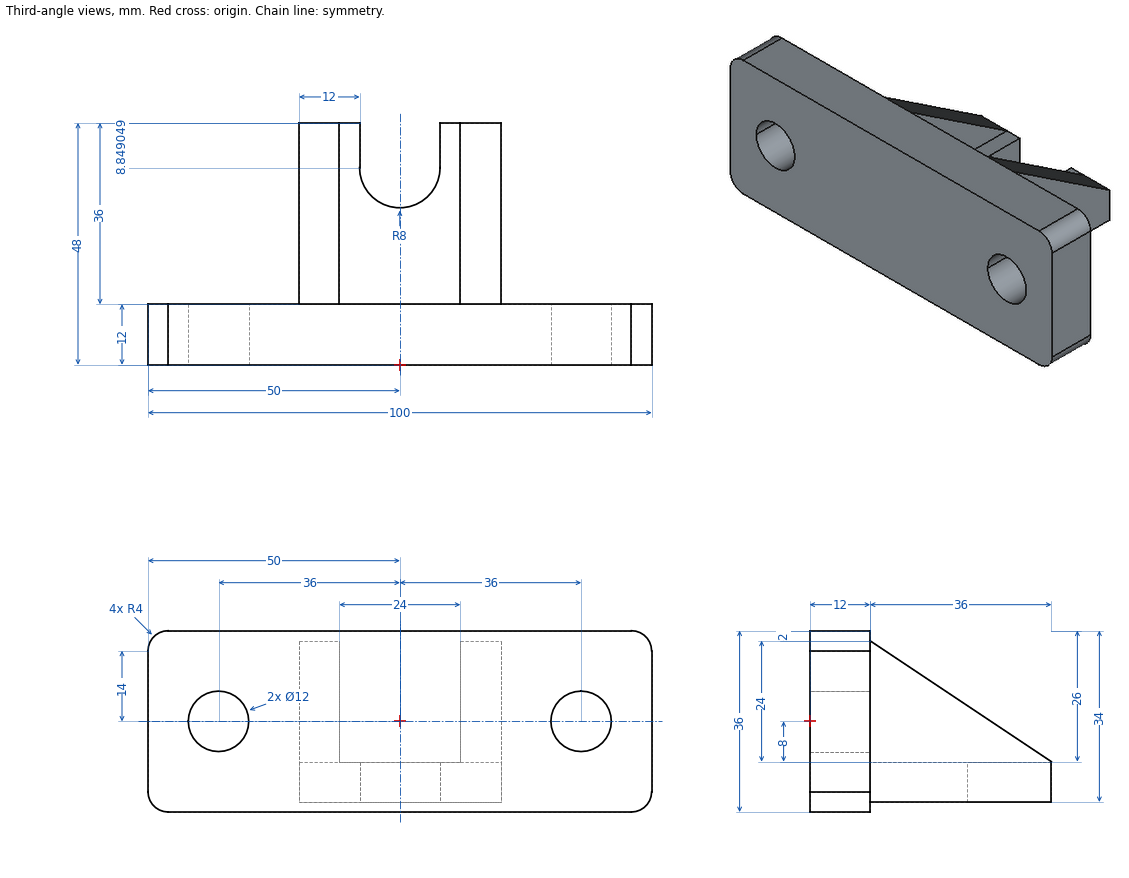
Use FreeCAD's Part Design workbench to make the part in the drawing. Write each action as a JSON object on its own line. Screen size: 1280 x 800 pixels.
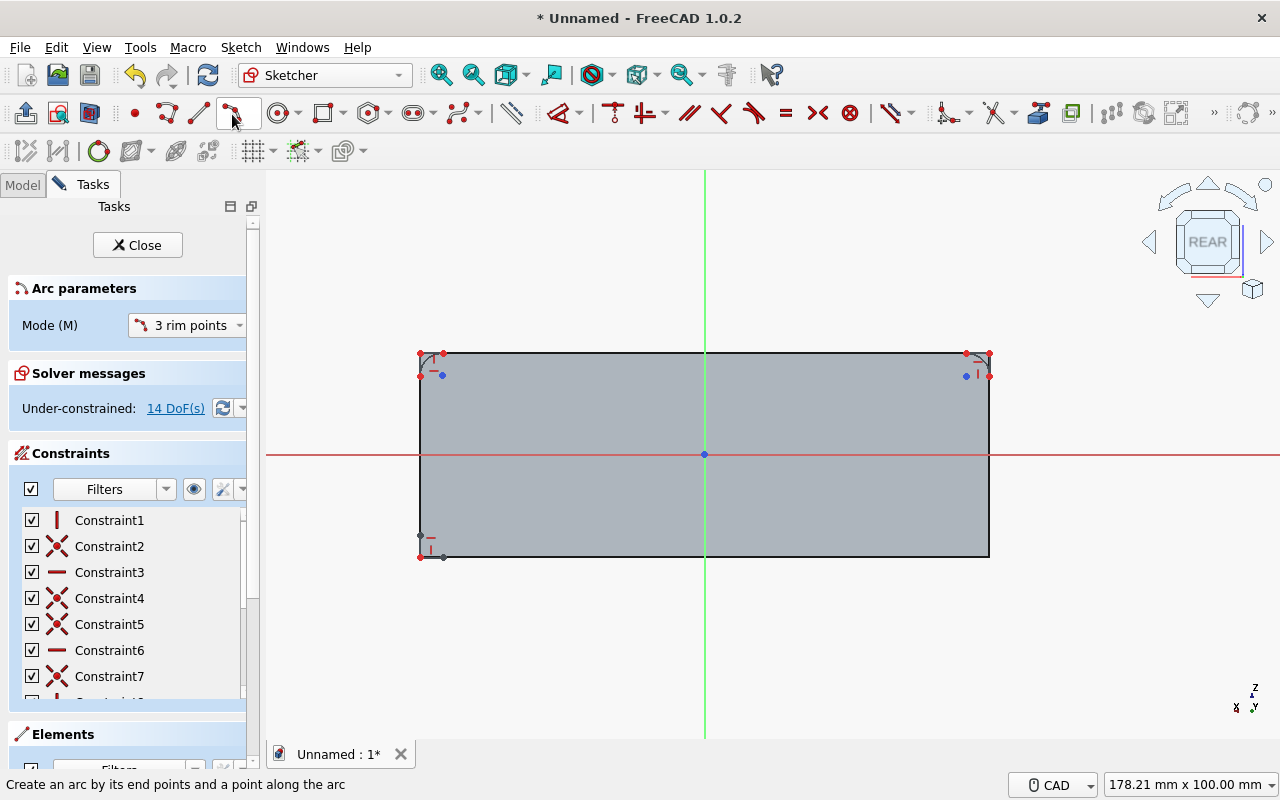
{"action": "scroll", "coordinate": [443, 557], "scroll_direction": "up", "scroll_amount": 2}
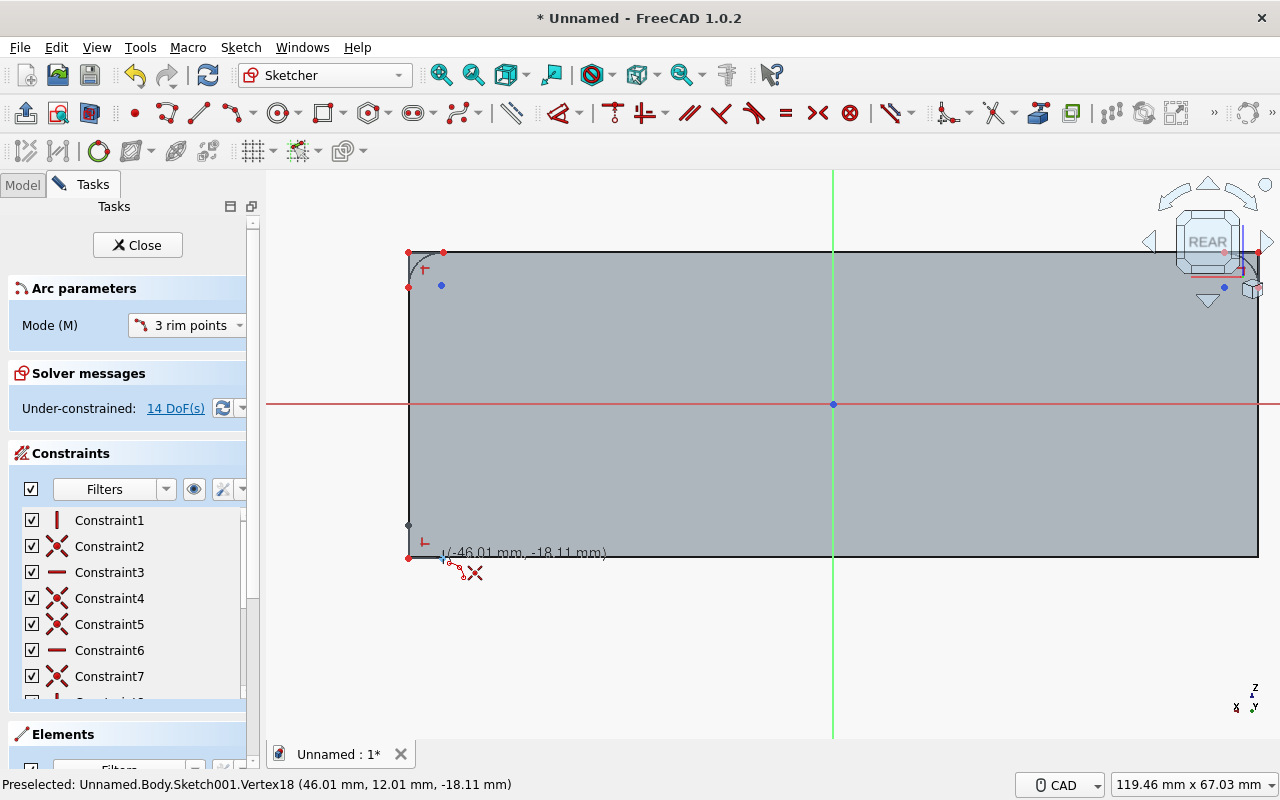
{"action": "left_click", "coordinate": [443, 558]}
{"action": "left_click", "coordinate": [409, 525]}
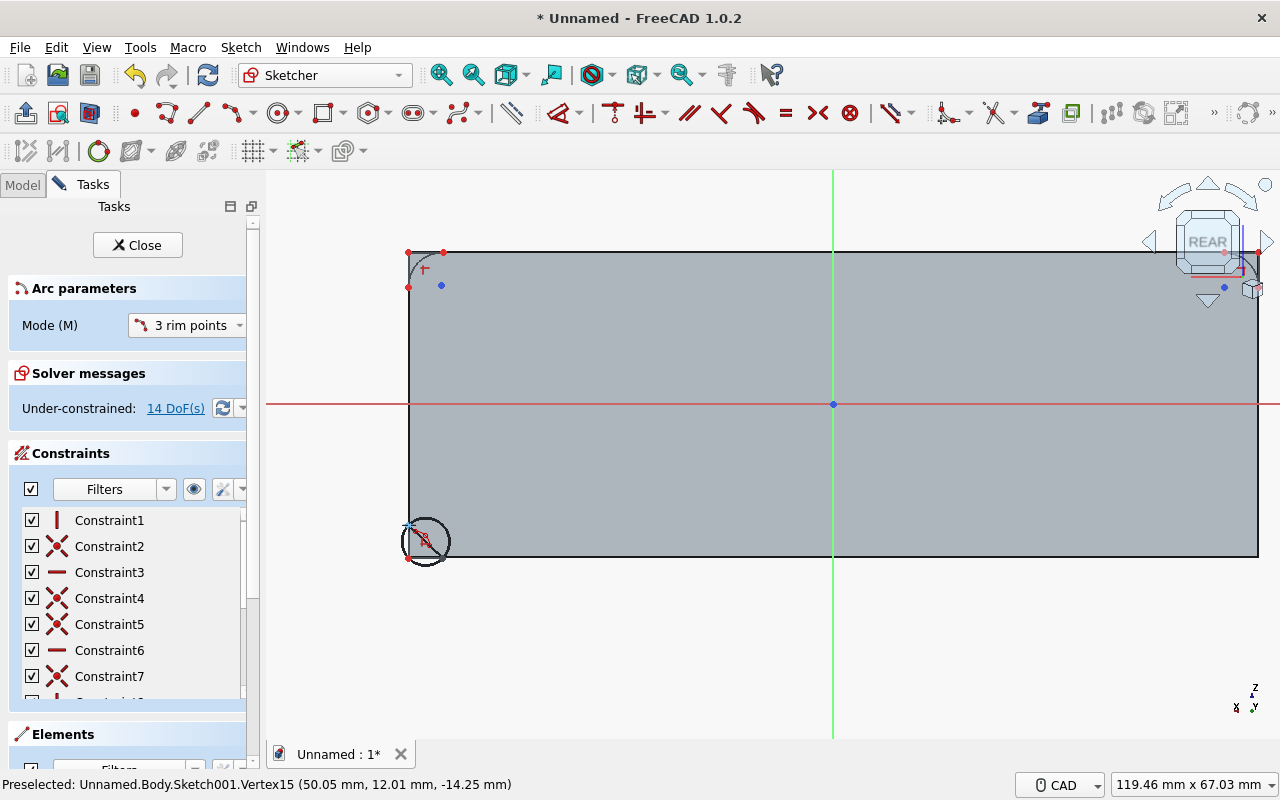
{"action": "scroll", "coordinate": [419, 547], "scroll_direction": "up", "scroll_amount": 3}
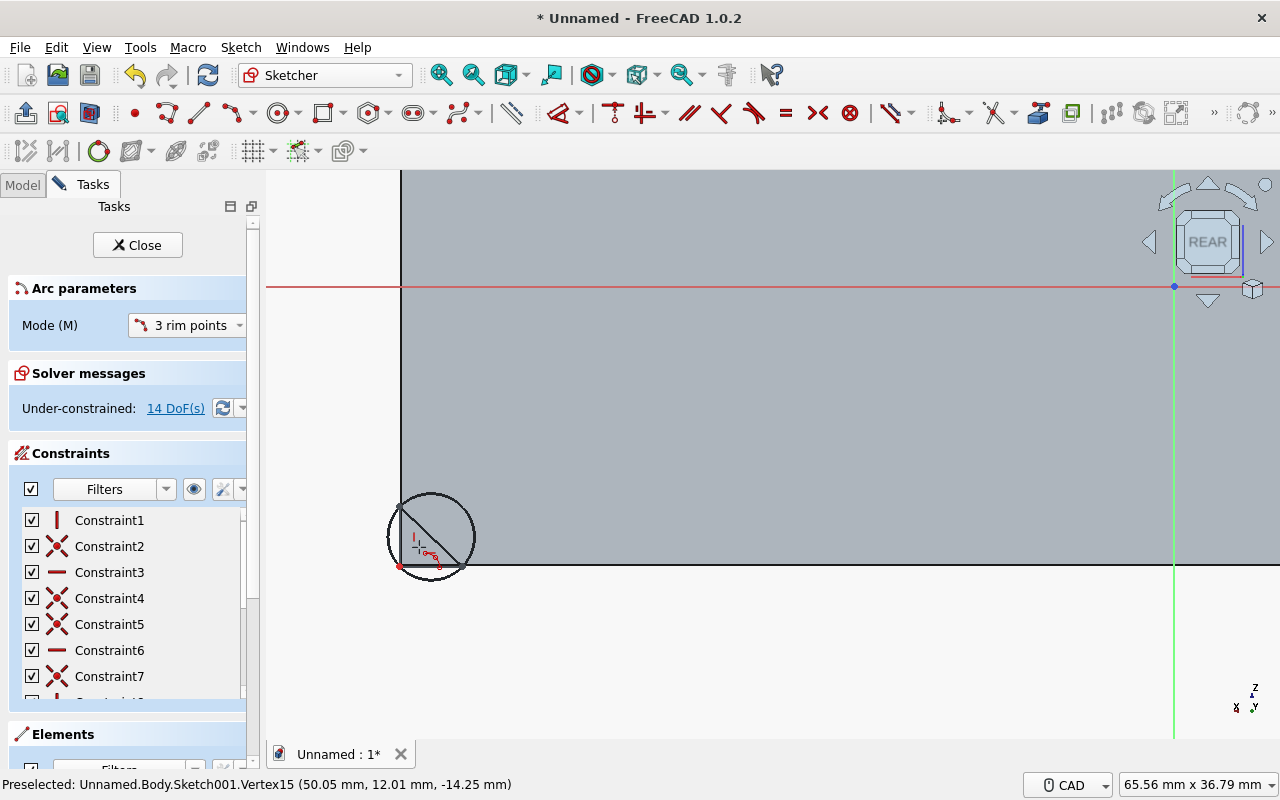
{"action": "left_click", "coordinate": [419, 547]}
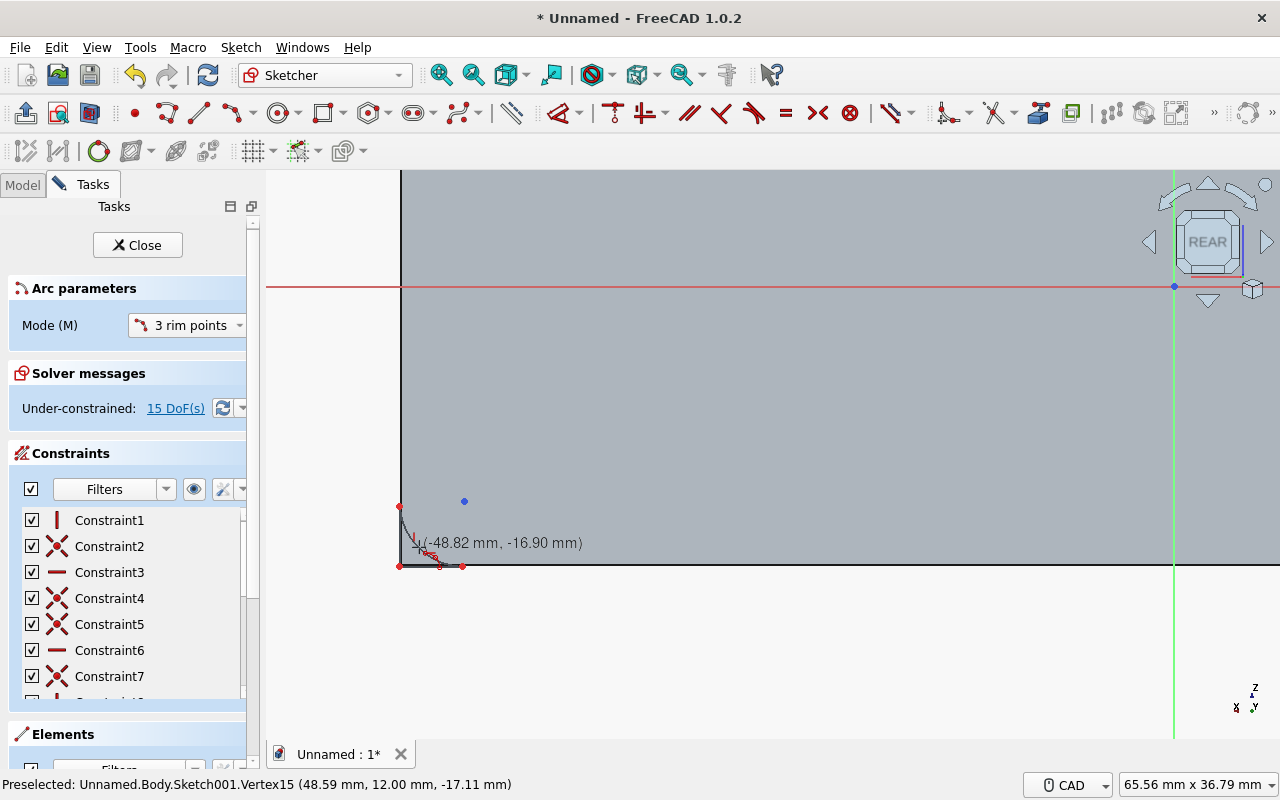
{"action": "left_click", "coordinate": [168, 114]}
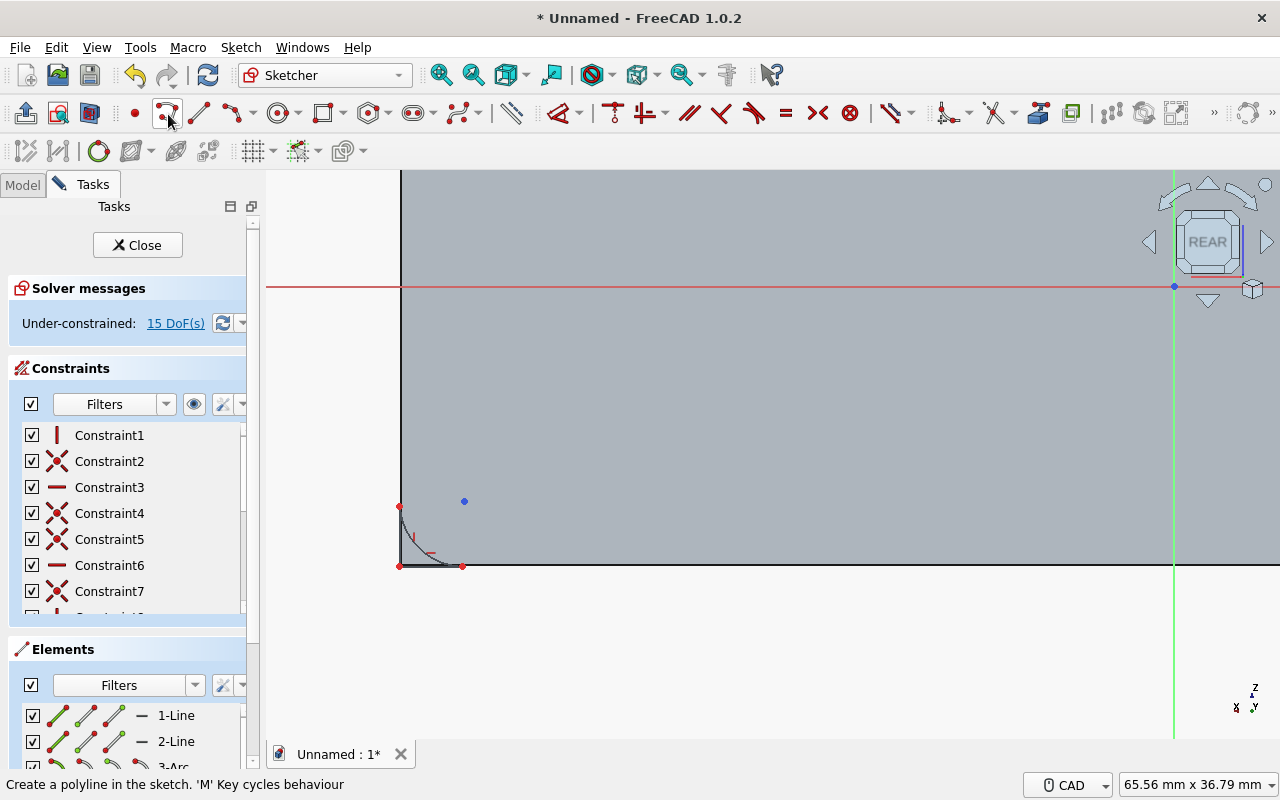
{"action": "scroll", "coordinate": [431, 552], "scroll_direction": "down", "scroll_amount": 5}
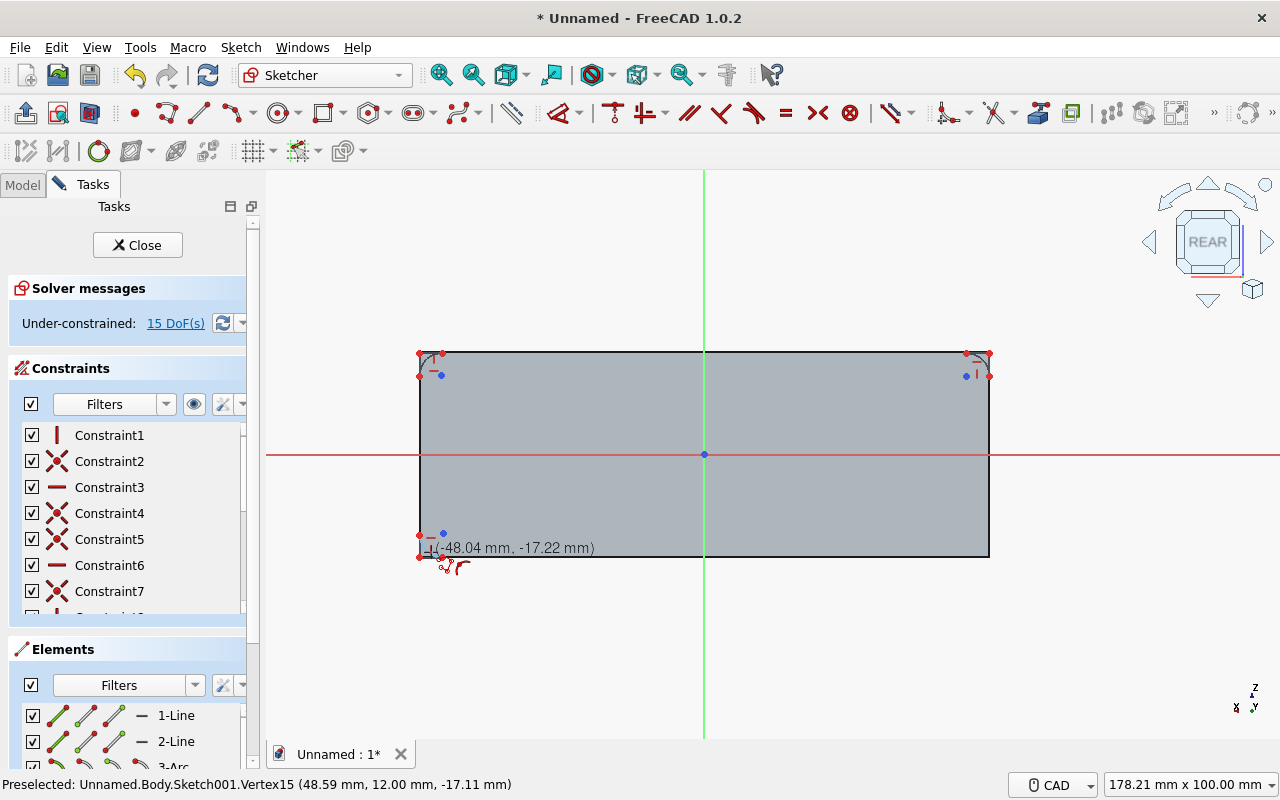
{"action": "left_click", "coordinate": [966, 557]}
{"action": "left_click", "coordinate": [989, 557]}
{"action": "left_click", "coordinate": [989, 534]}
{"action": "right_click", "coordinate": [989, 534]}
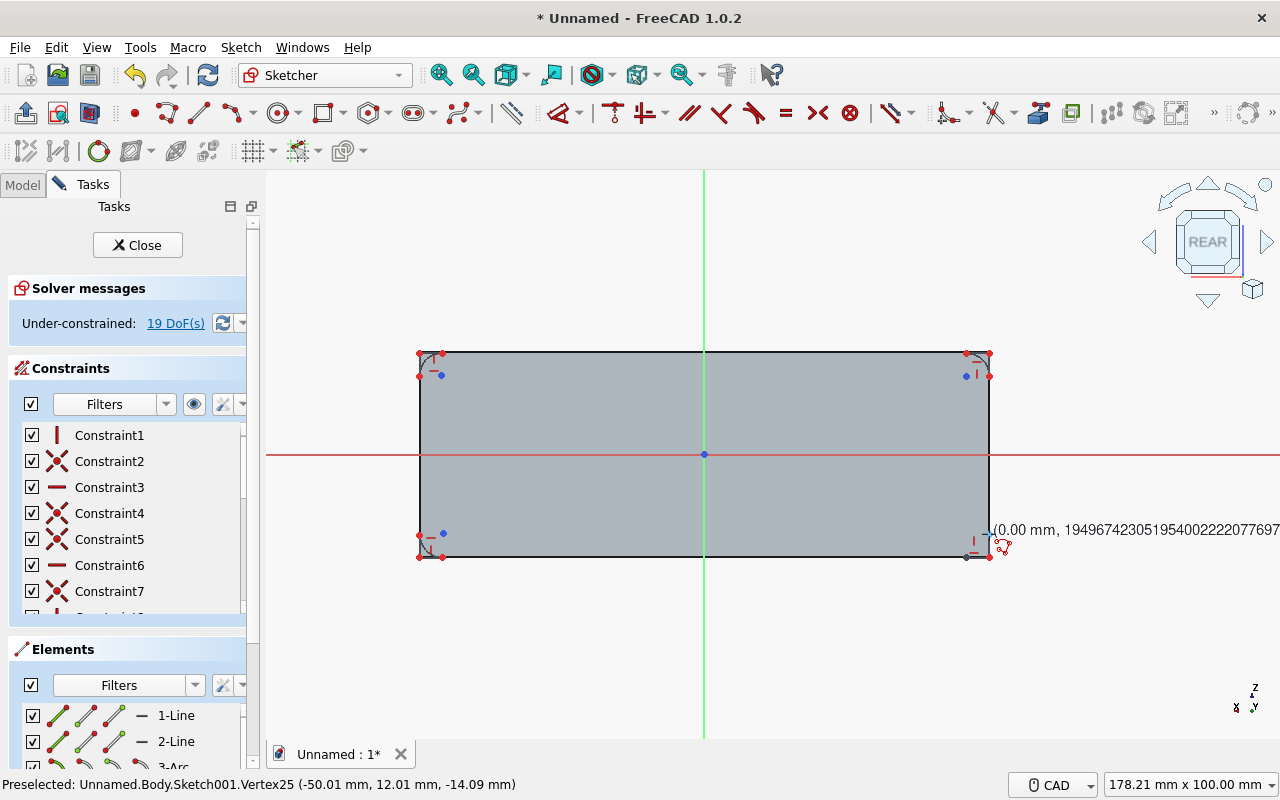
{"action": "left_click", "coordinate": [232, 114]}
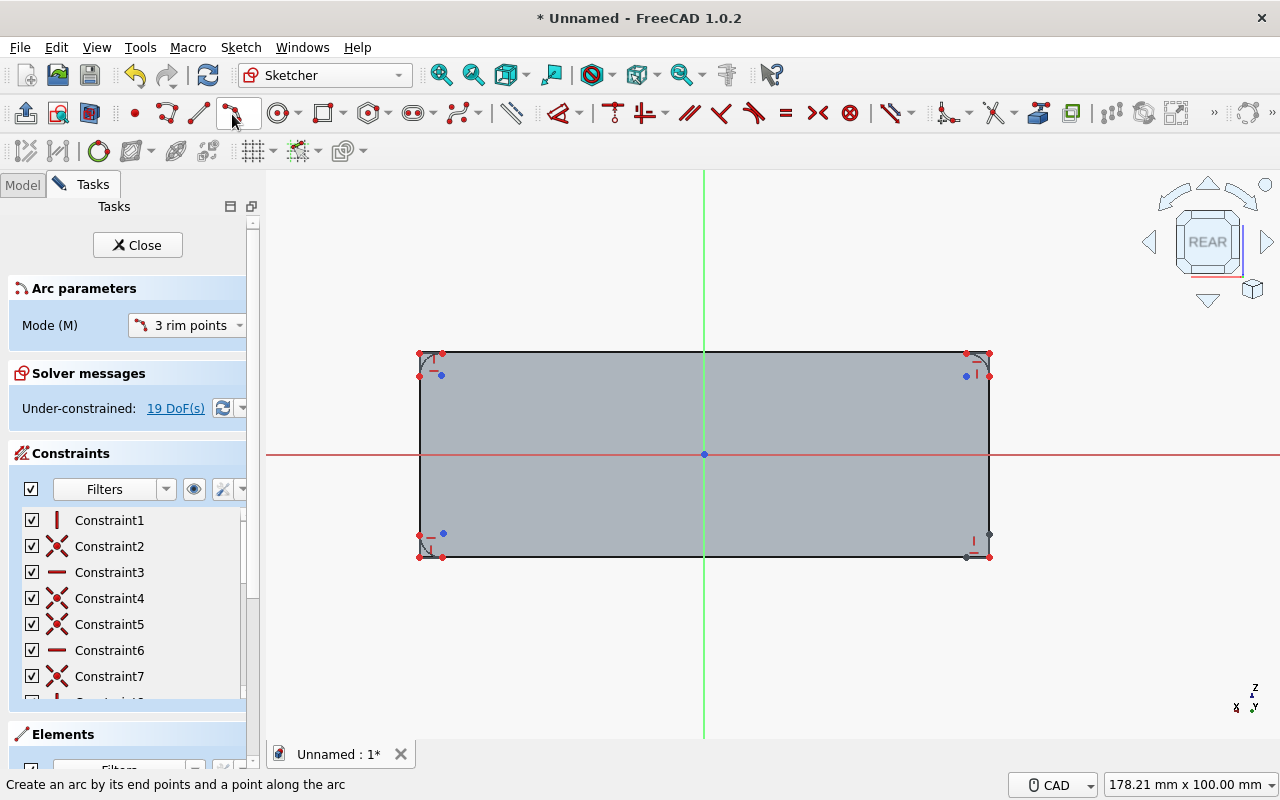
{"action": "scroll", "coordinate": [989, 534], "scroll_direction": "up", "scroll_amount": 2}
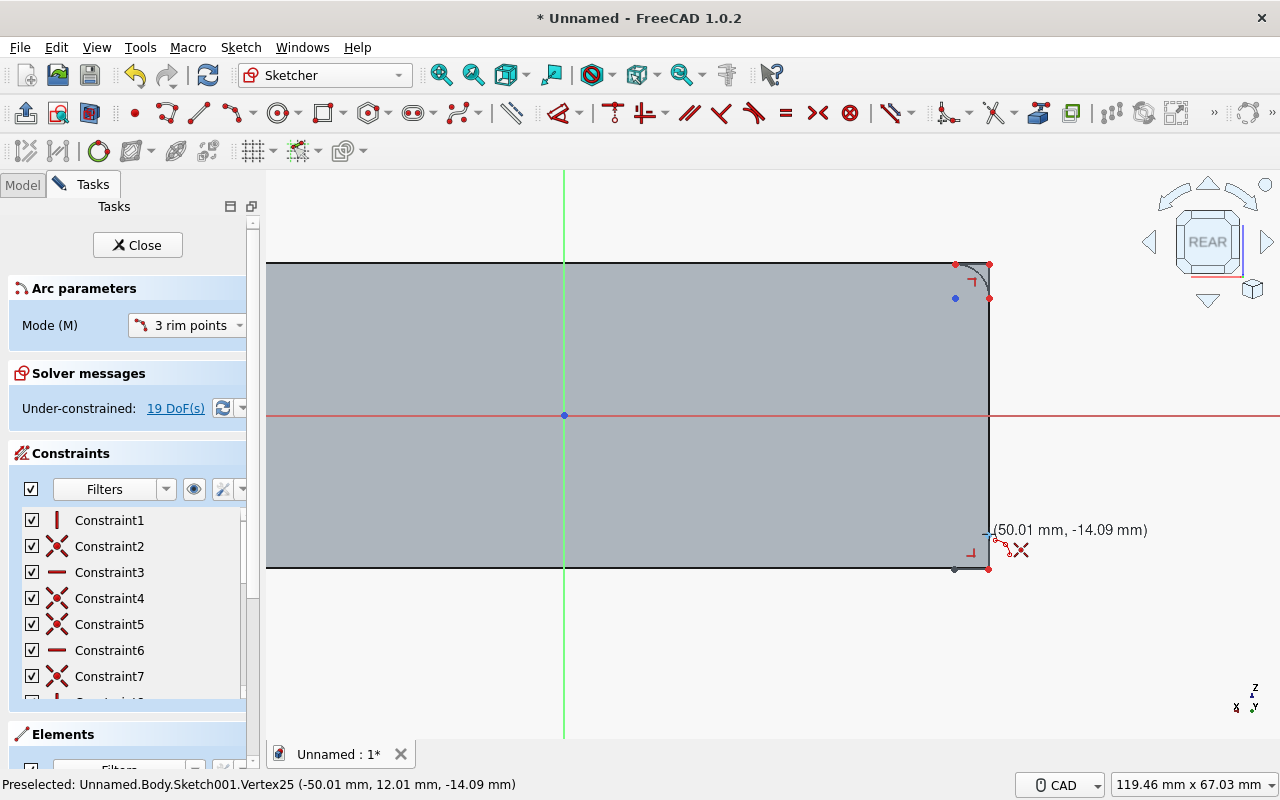
{"action": "left_click", "coordinate": [989, 535]}
{"action": "left_click", "coordinate": [954, 569]}